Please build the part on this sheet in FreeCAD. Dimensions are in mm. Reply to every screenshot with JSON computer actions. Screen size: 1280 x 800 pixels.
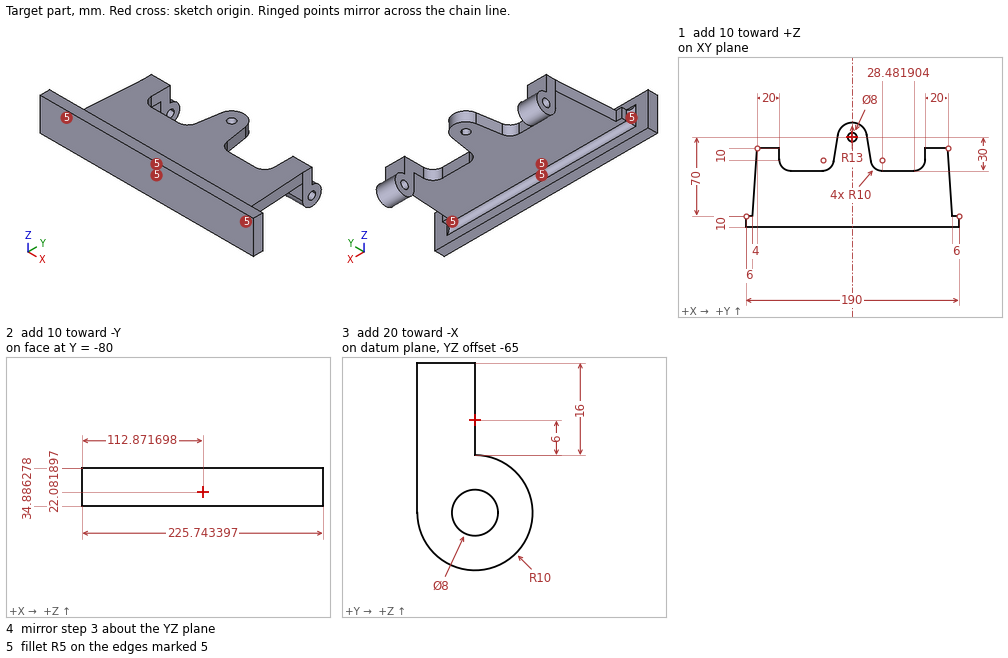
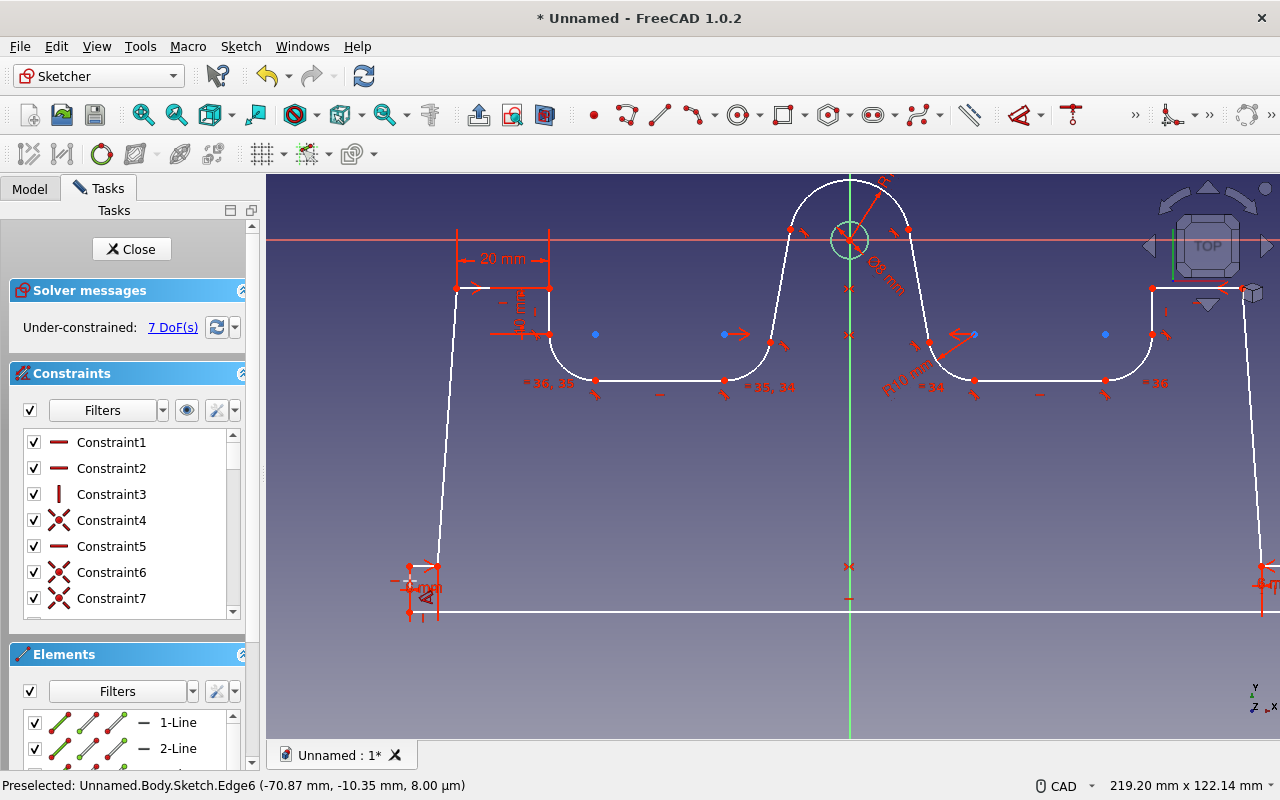
{"action": "left_click", "coordinate": [410, 580]}
{"action": "left_click", "coordinate": [352, 589]}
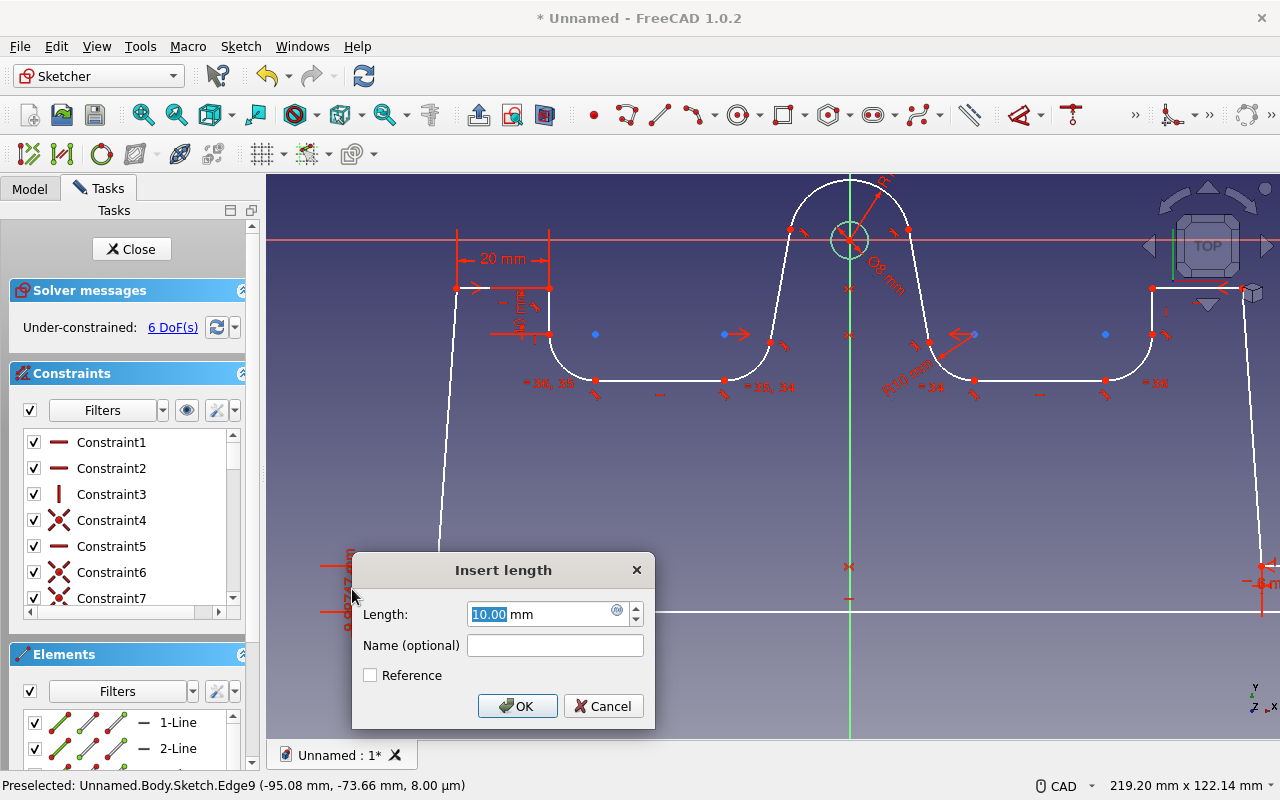
{"action": "type", "text": "10"}
{"action": "key", "text": "Return"}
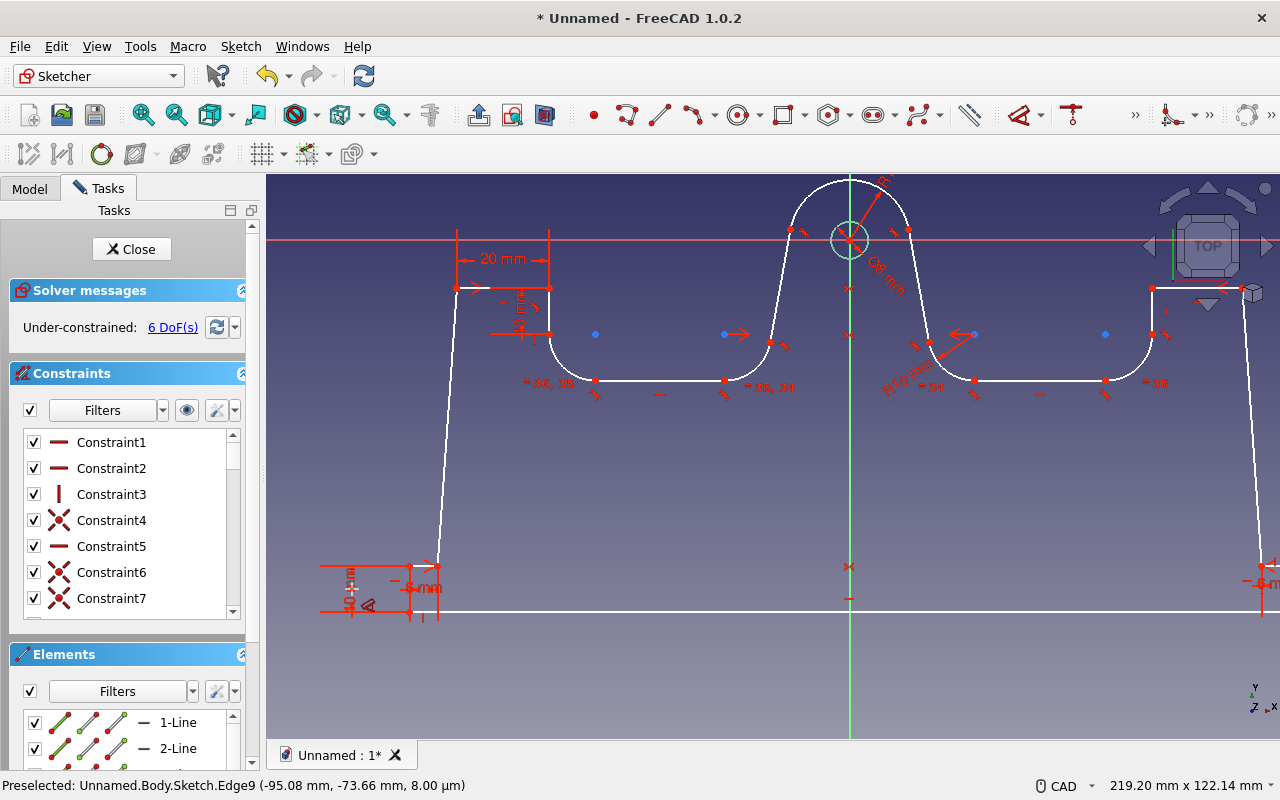
{"action": "scroll", "coordinate": [409, 581], "scroll_direction": "down", "scroll_amount": 2}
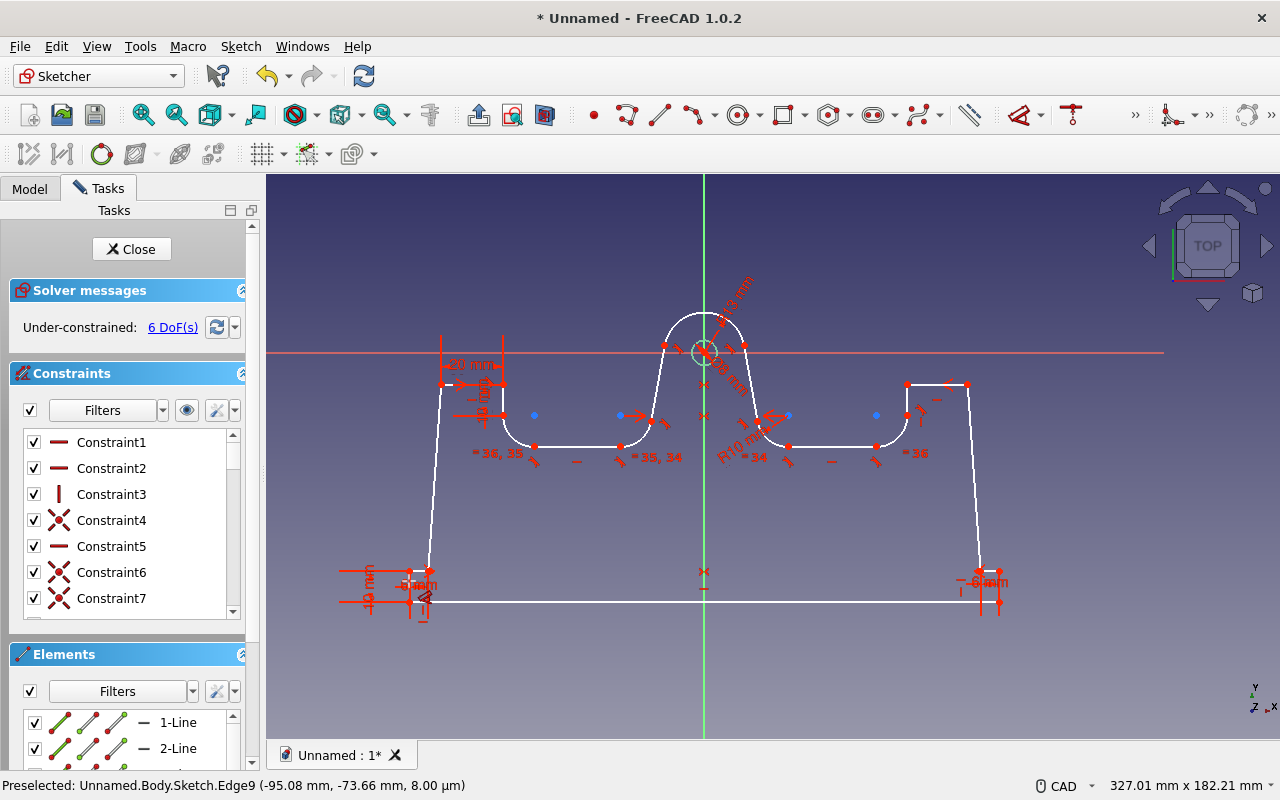
{"action": "left_click", "coordinate": [950, 385]}
{"action": "left_click", "coordinate": [937, 419]}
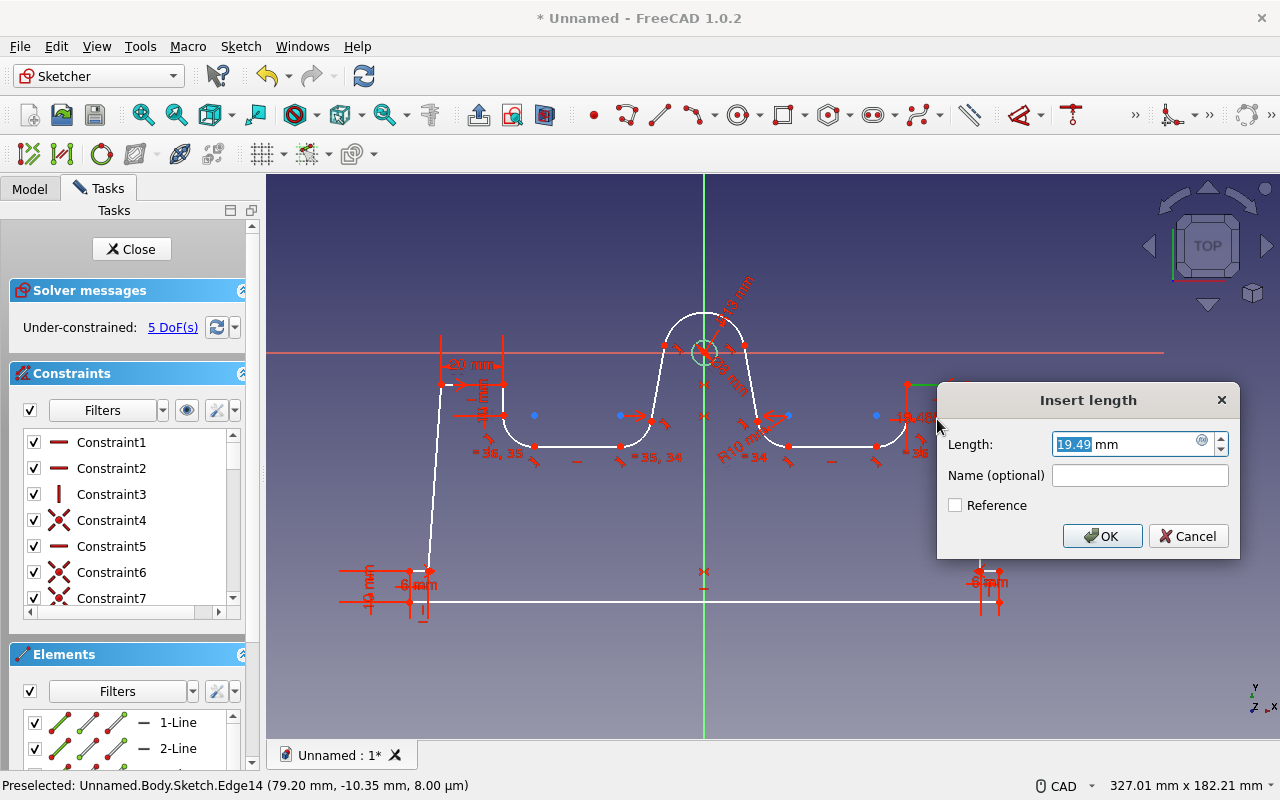
{"action": "type", "text": "20"}
{"action": "key", "text": "Return"}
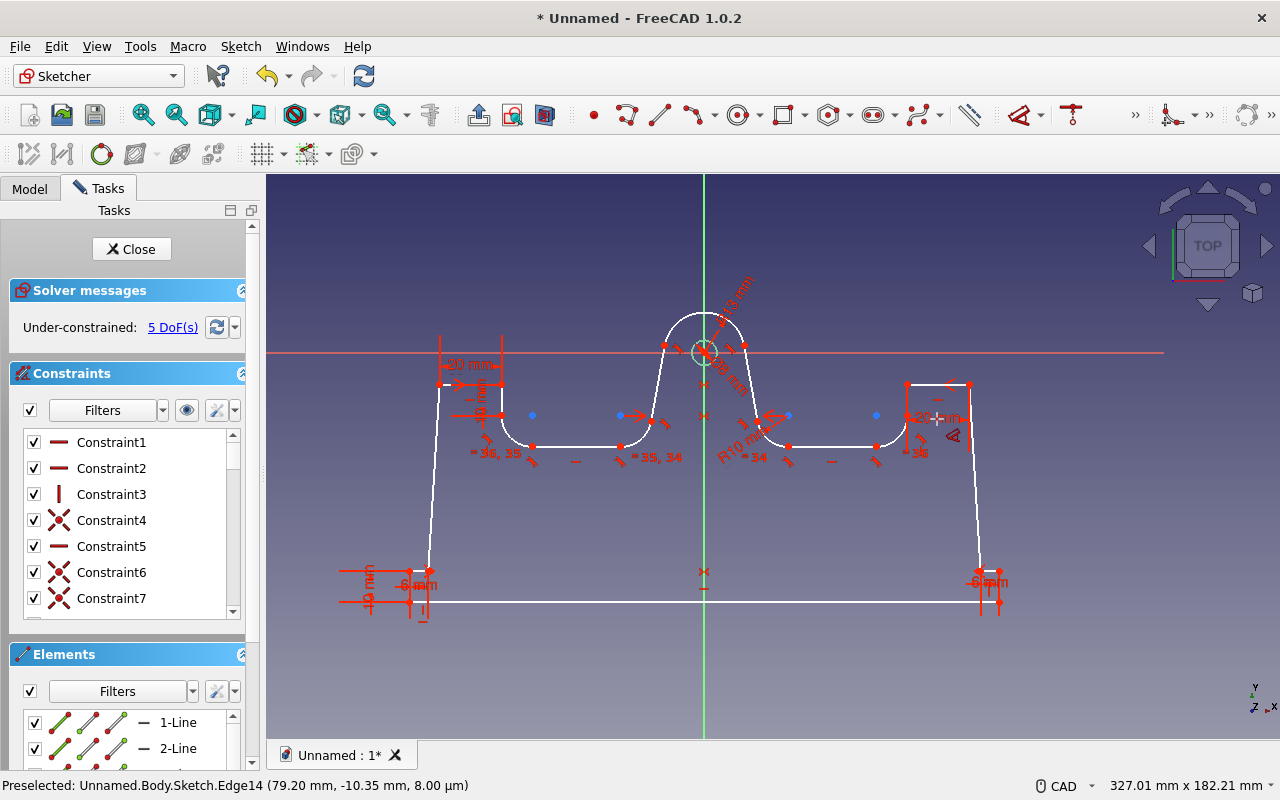
{"action": "scroll", "coordinate": [436, 441], "scroll_direction": "up", "scroll_amount": 6}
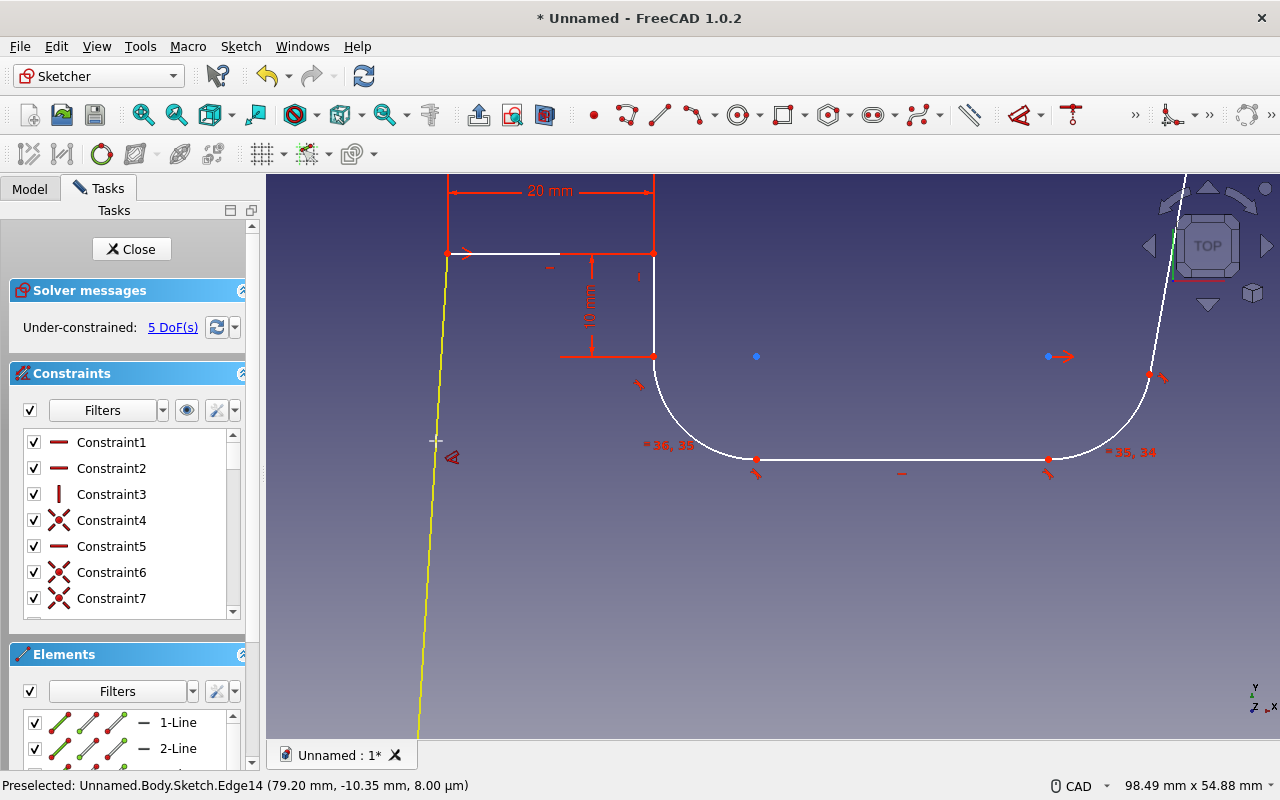
{"action": "left_click", "coordinate": [436, 439]}
{"action": "left_click", "coordinate": [429, 220]}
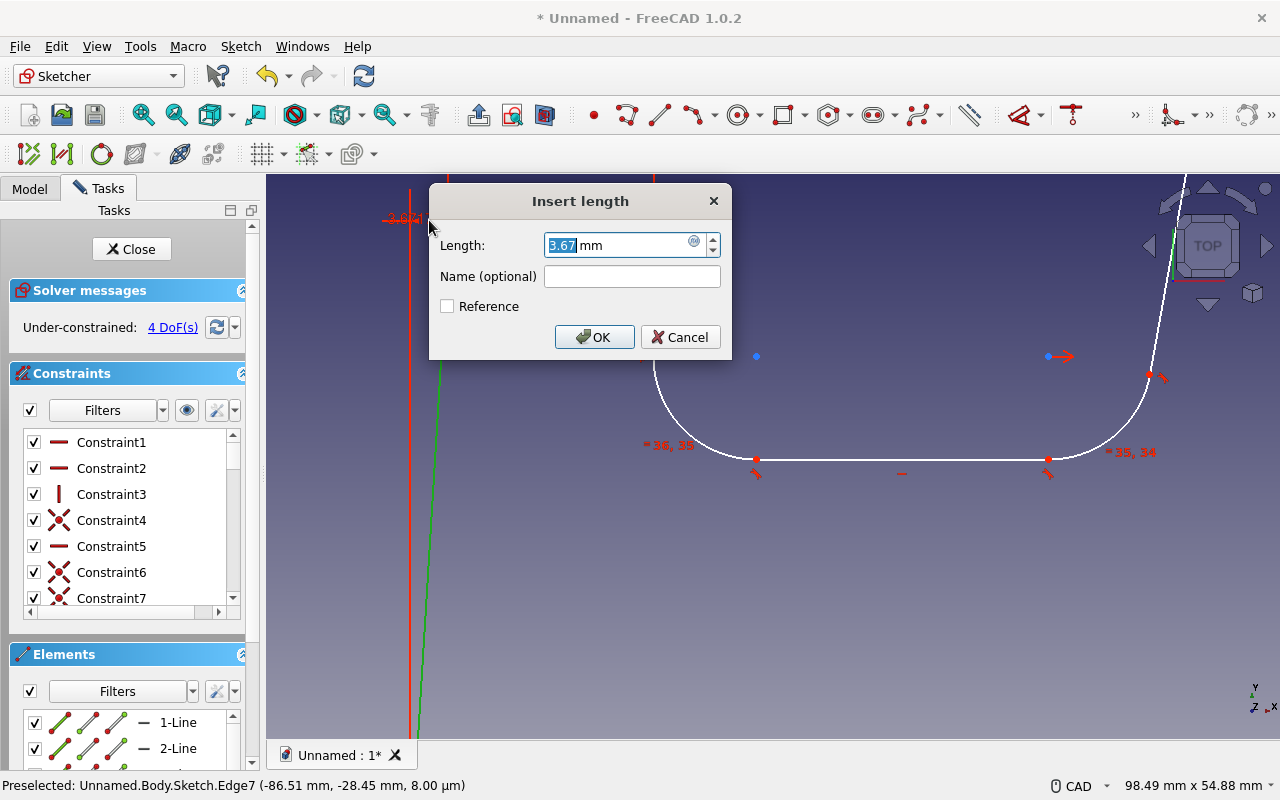
{"action": "type", "text": "4"}
{"action": "key", "text": "Return"}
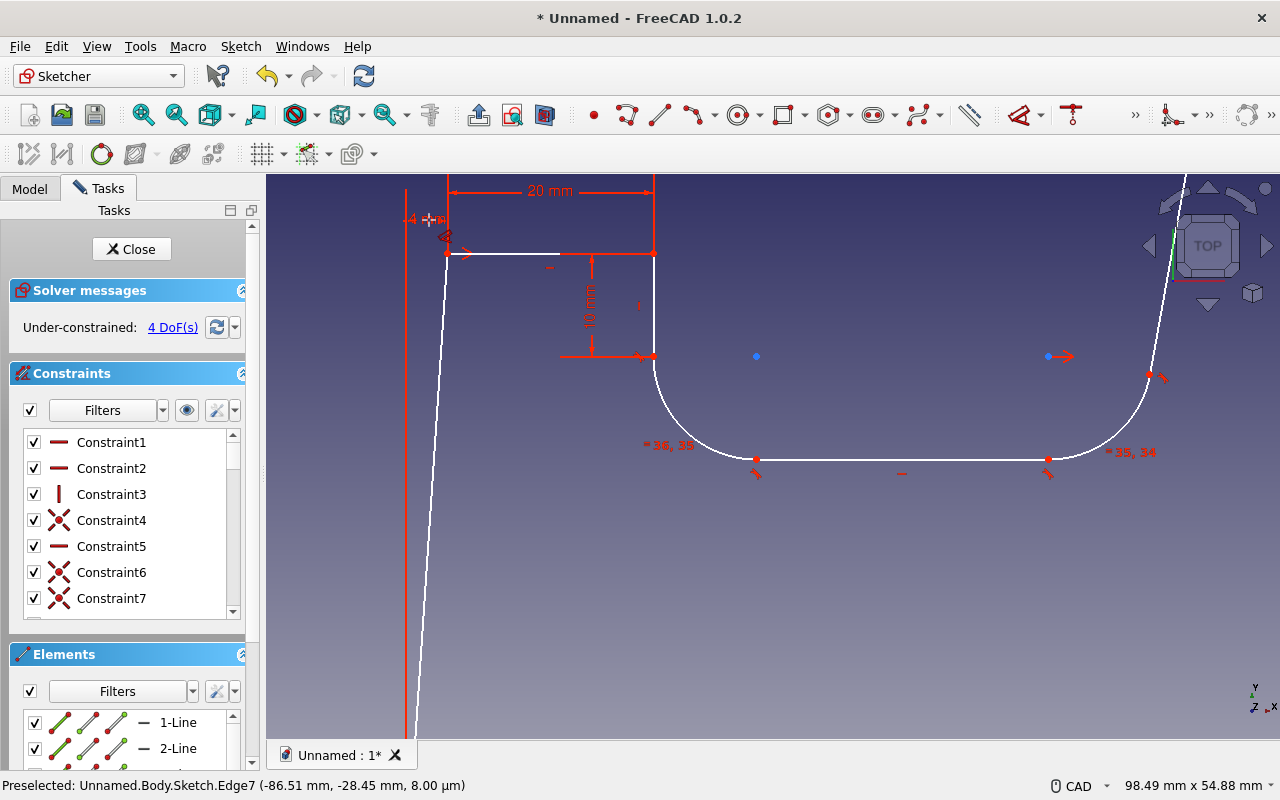
{"action": "scroll", "coordinate": [436, 441], "scroll_direction": "down", "scroll_amount": 6}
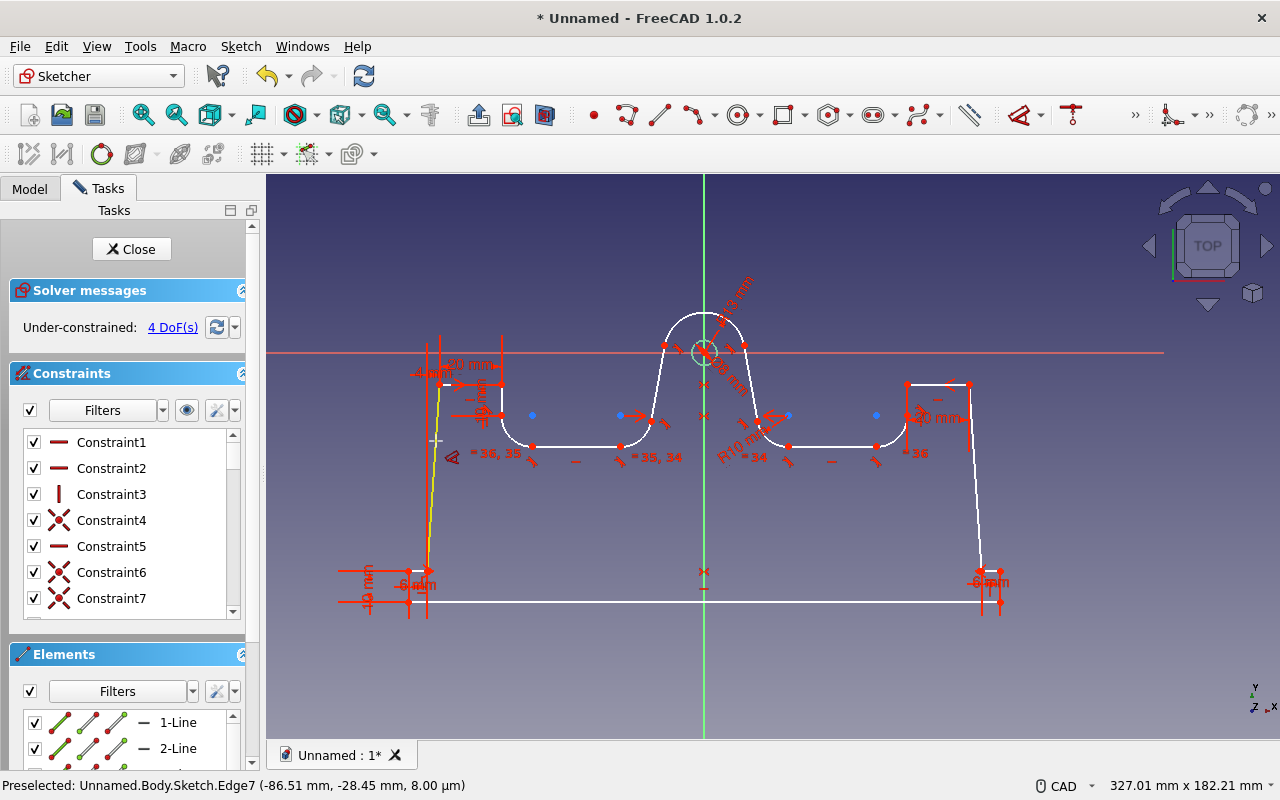
{"action": "left_click", "coordinate": [586, 602]}
{"action": "left_click", "coordinate": [568, 636]}